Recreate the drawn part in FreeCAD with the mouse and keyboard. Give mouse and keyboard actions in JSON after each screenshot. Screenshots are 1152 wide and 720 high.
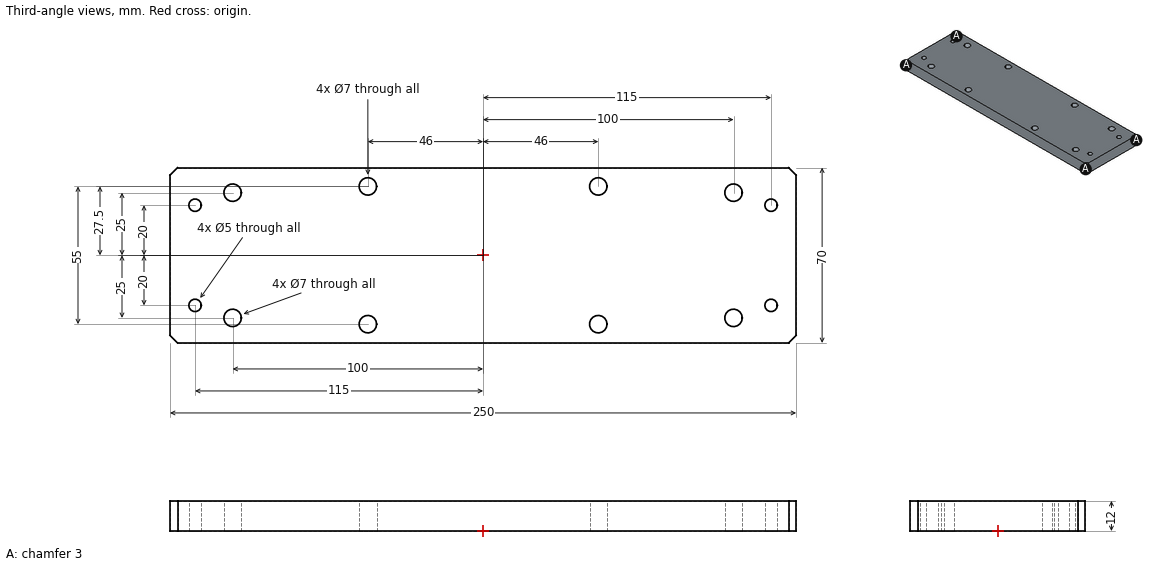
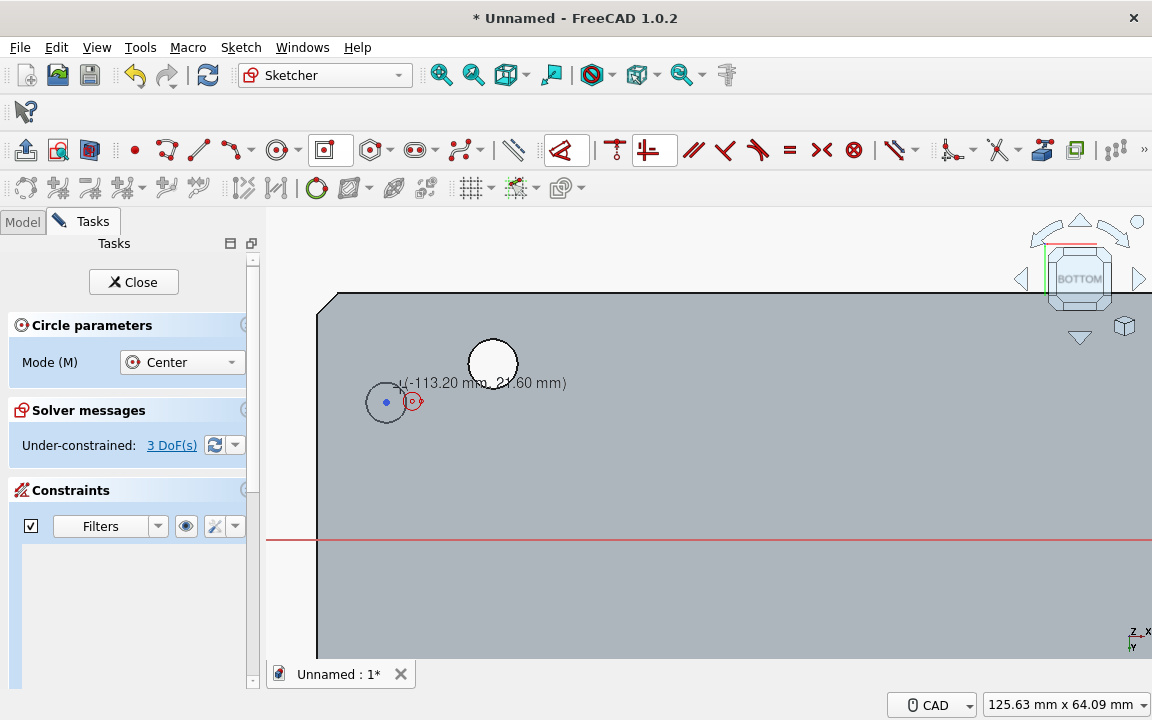
{"action": "scroll", "coordinate": [400, 387], "scroll_direction": "down", "scroll_amount": 6}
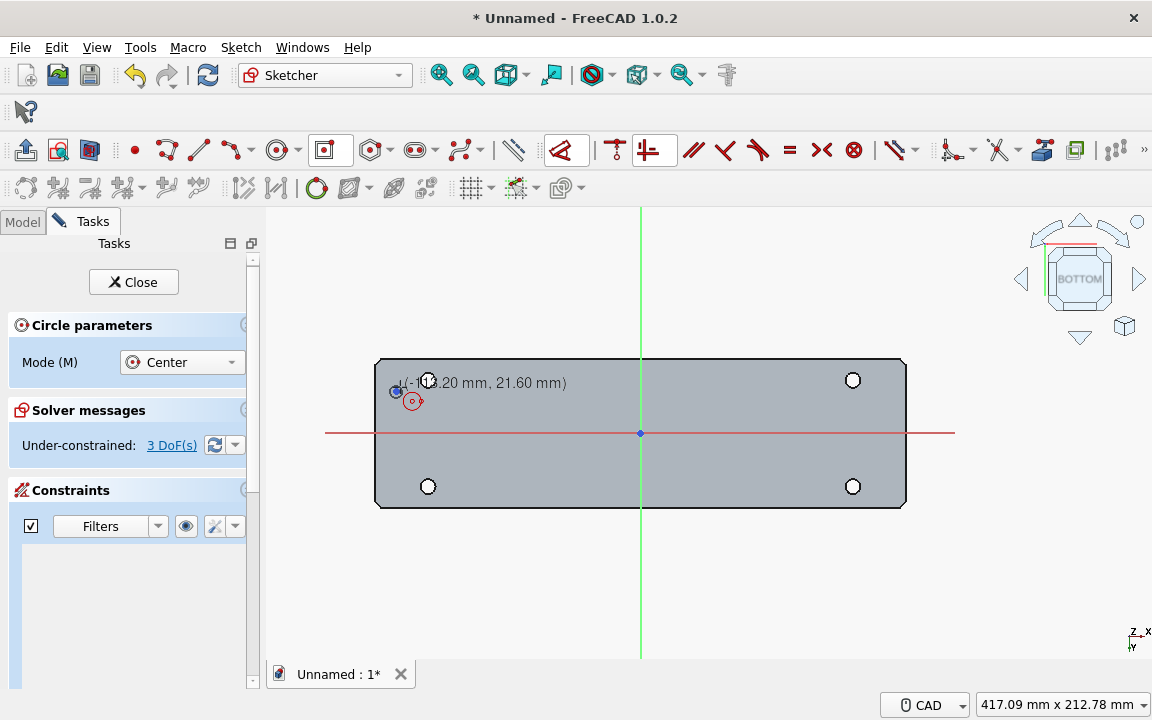
{"action": "scroll", "coordinate": [396, 476], "scroll_direction": "up", "scroll_amount": 8}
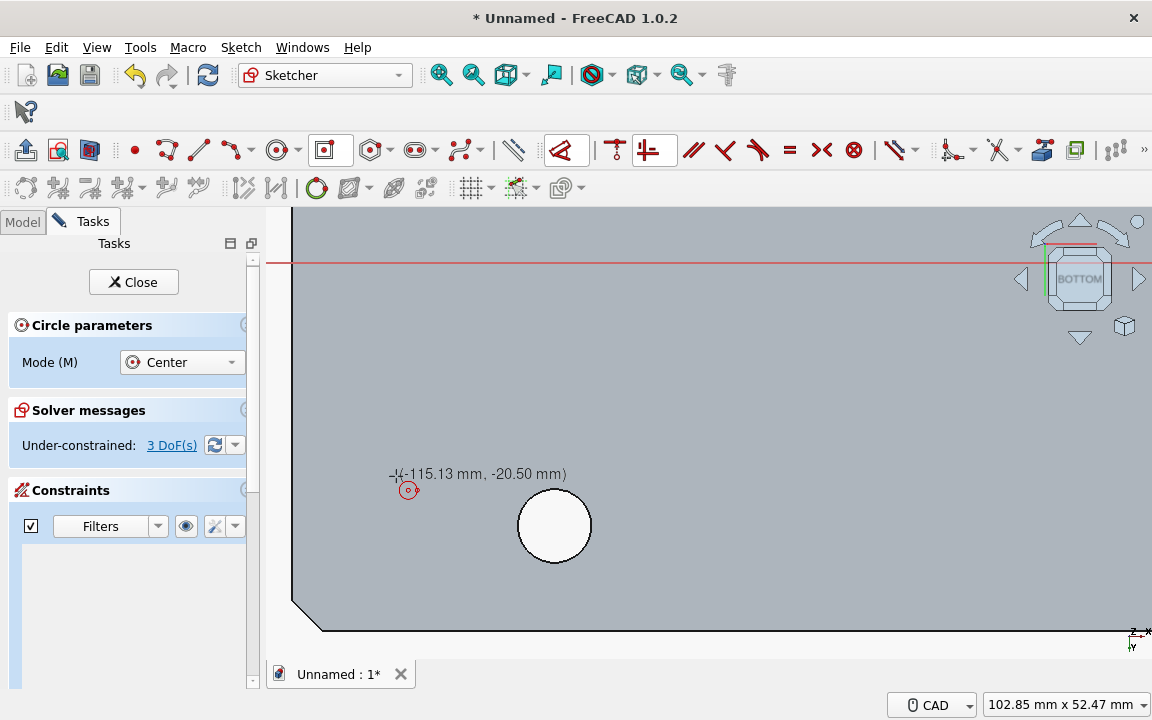
{"action": "scroll", "coordinate": [396, 476], "scroll_direction": "down", "scroll_amount": 8}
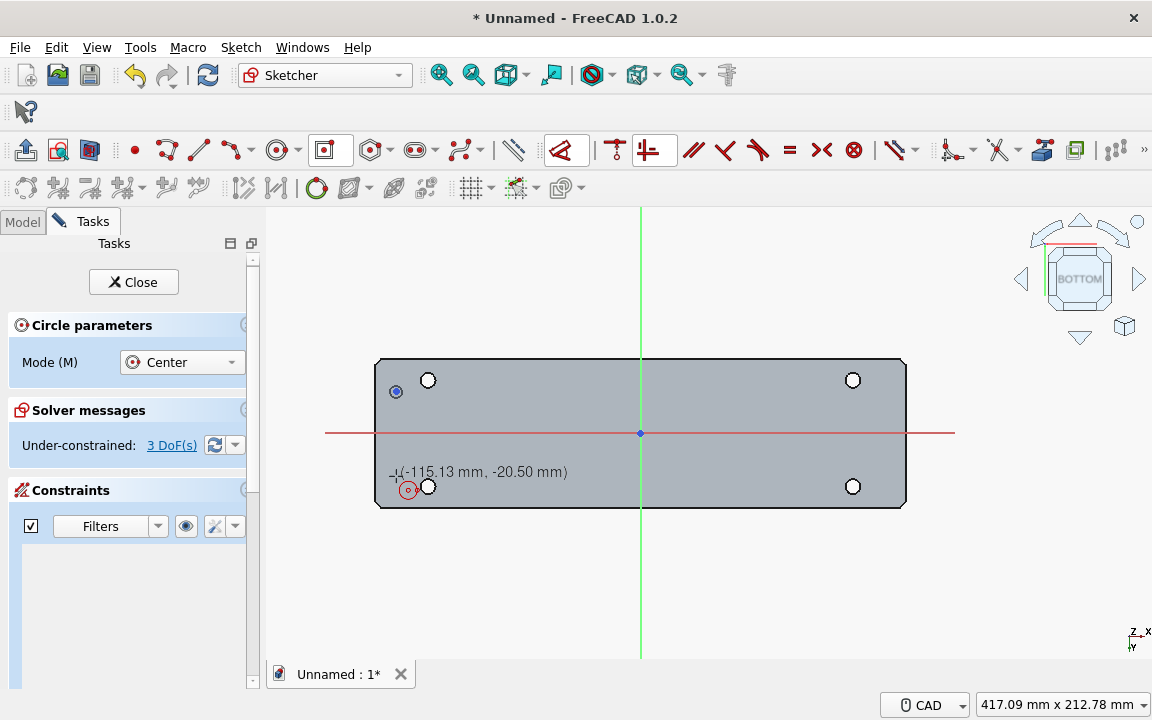
{"action": "left_click", "coordinate": [396, 476]}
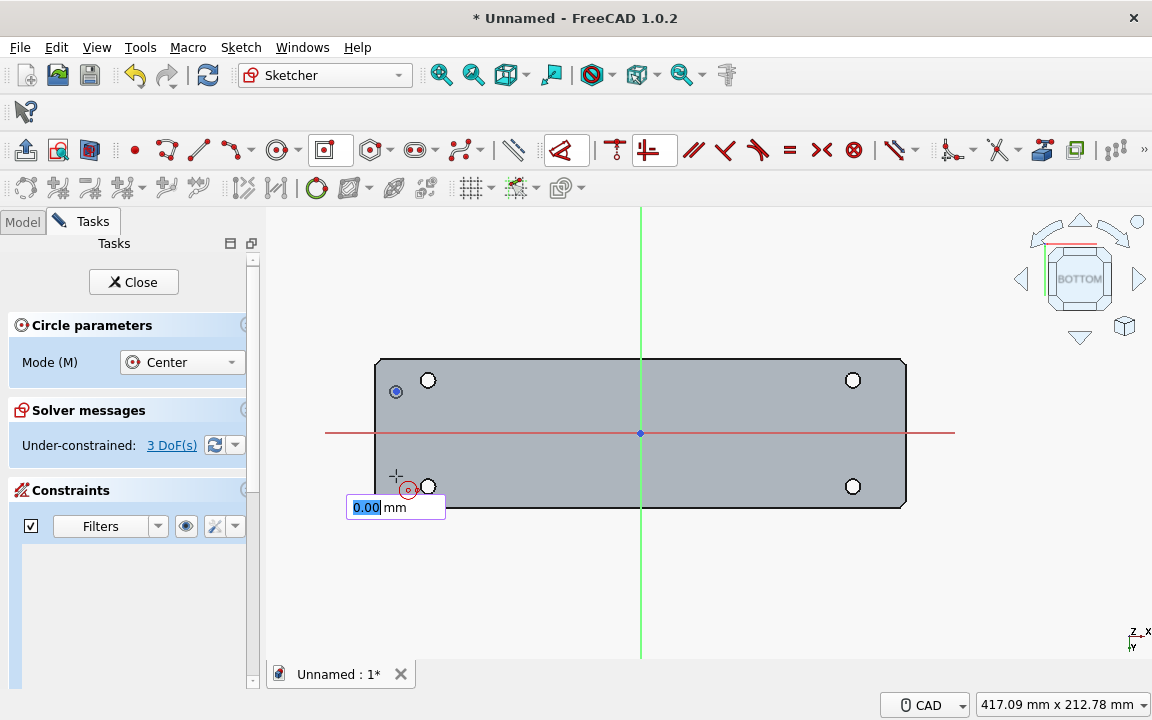
{"action": "scroll", "coordinate": [400, 472], "scroll_direction": "up", "scroll_amount": 6}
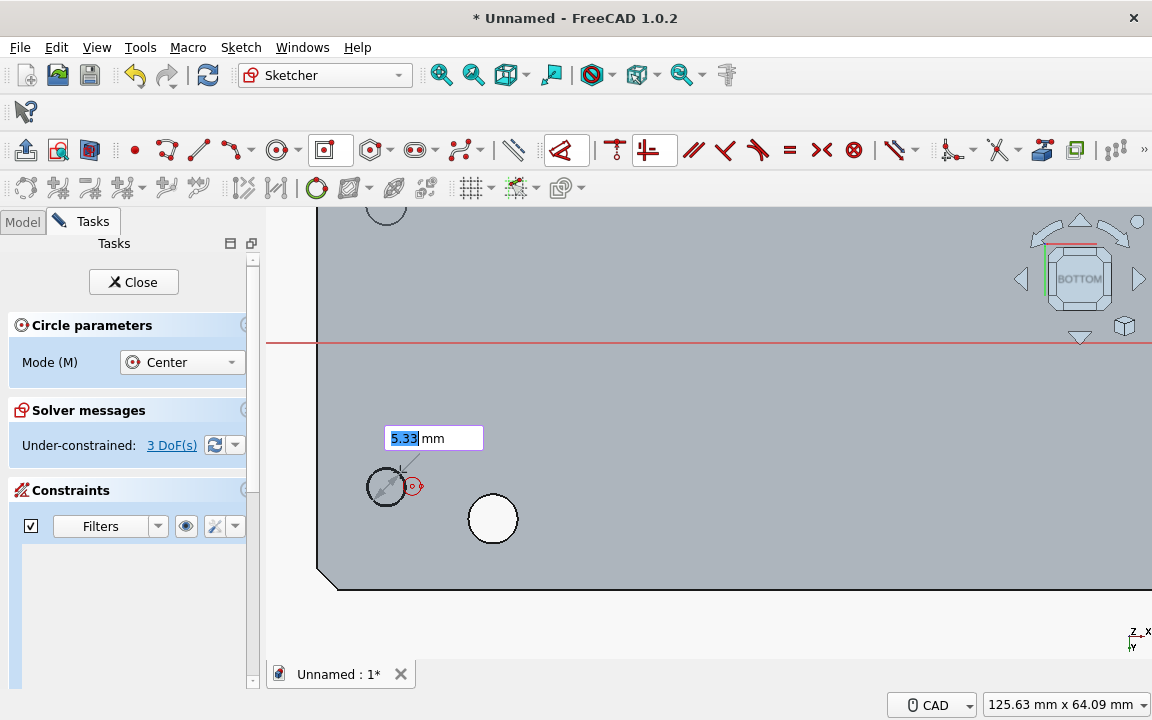
{"action": "left_click", "coordinate": [400, 471]}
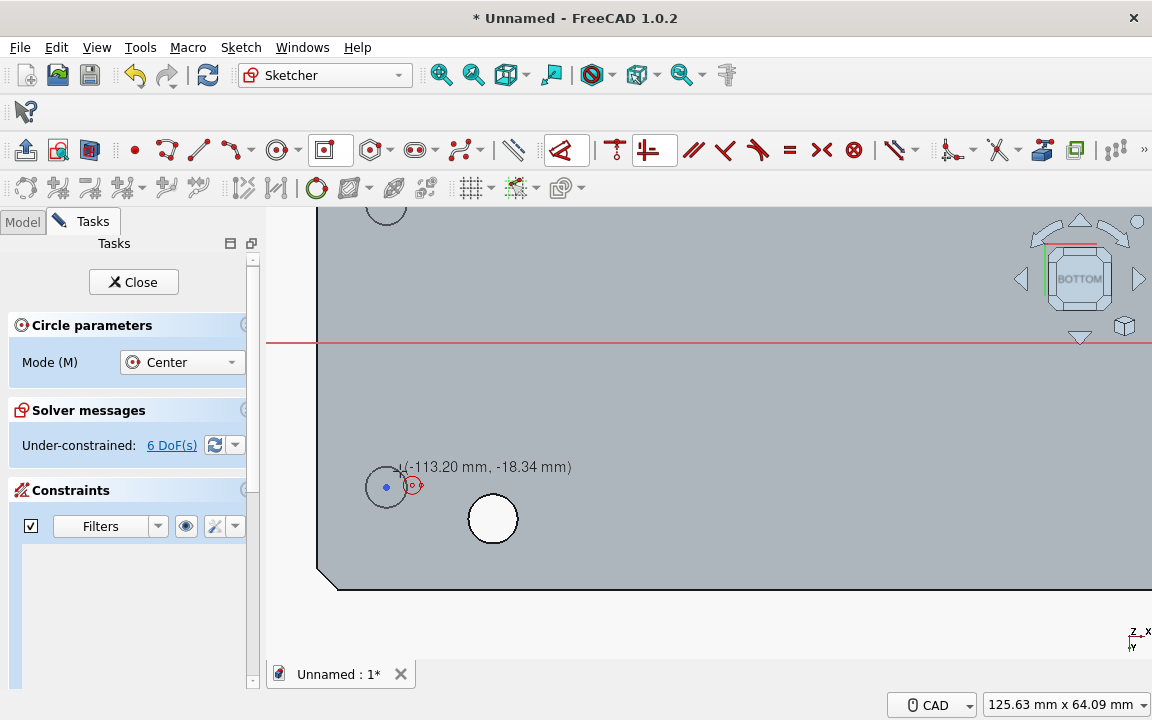
{"action": "scroll", "coordinate": [400, 472], "scroll_direction": "down", "scroll_amount": 6}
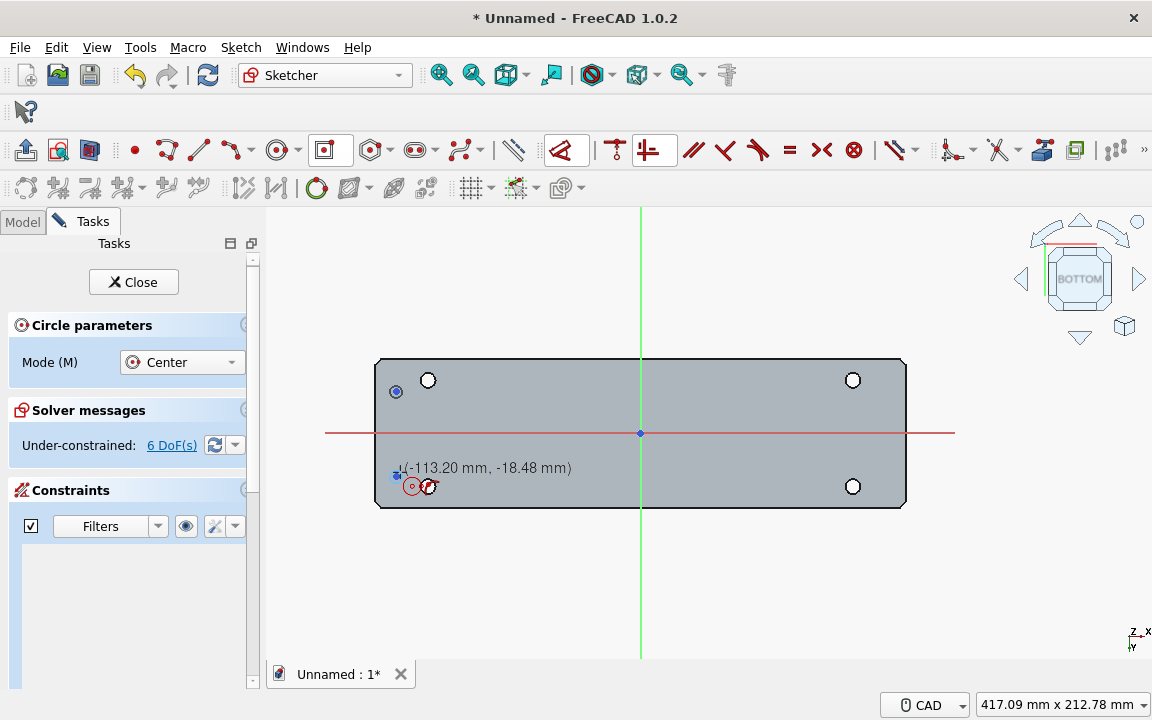
{"action": "scroll", "coordinate": [885, 476], "scroll_direction": "up", "scroll_amount": 8}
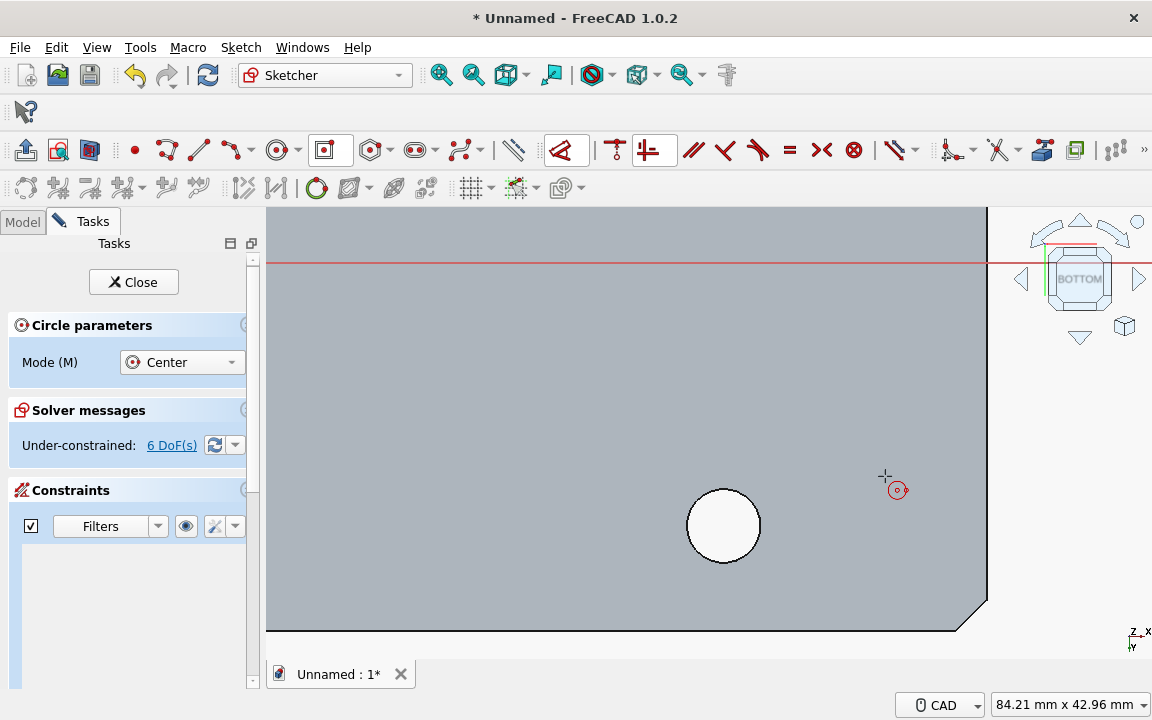
{"action": "scroll", "coordinate": [886, 476], "scroll_direction": "down", "scroll_amount": 8}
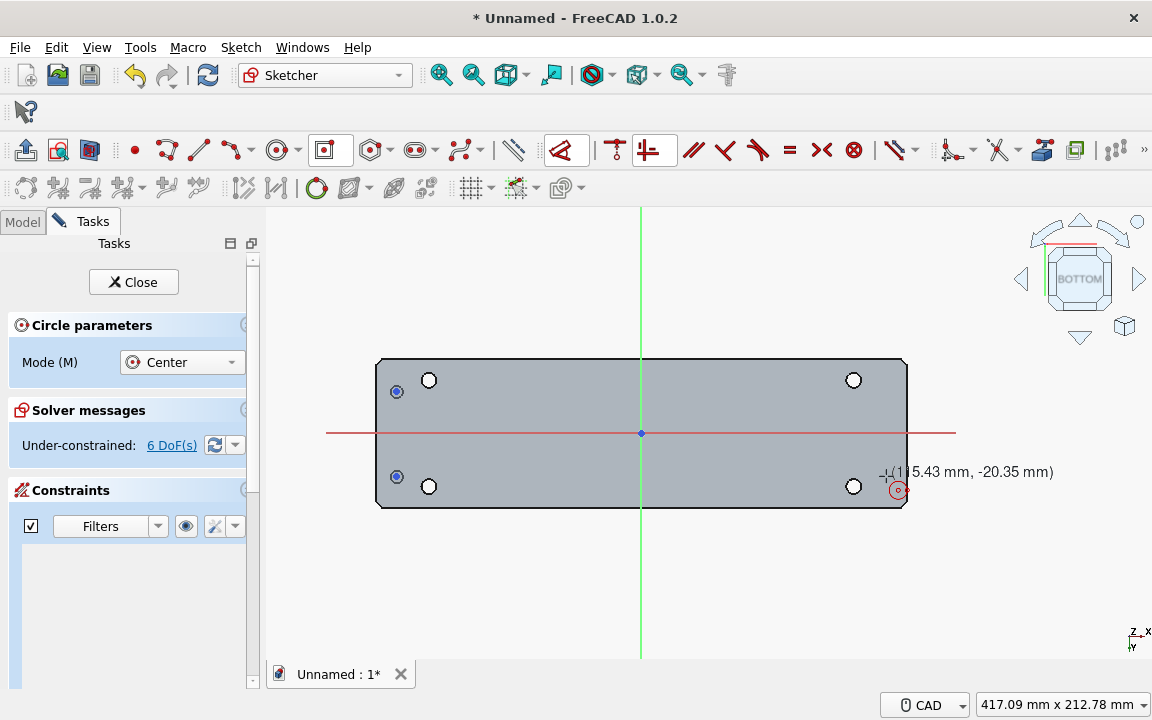
{"action": "left_click", "coordinate": [886, 476]}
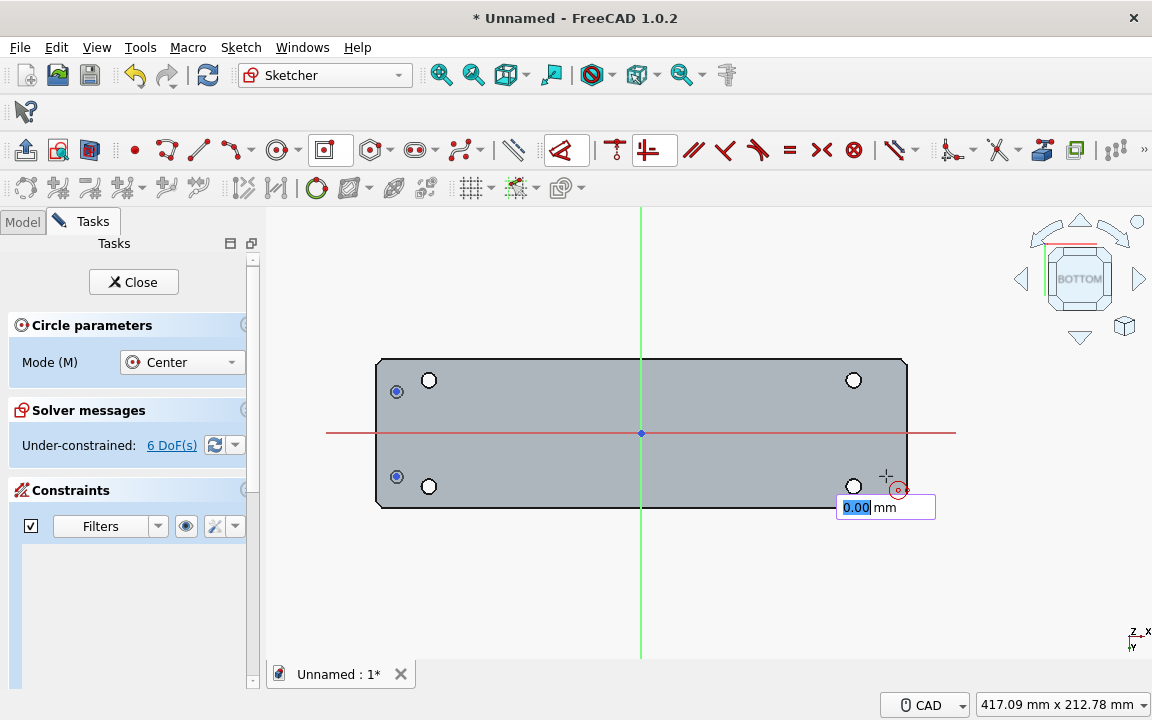
{"action": "scroll", "coordinate": [889, 472], "scroll_direction": "up", "scroll_amount": 6}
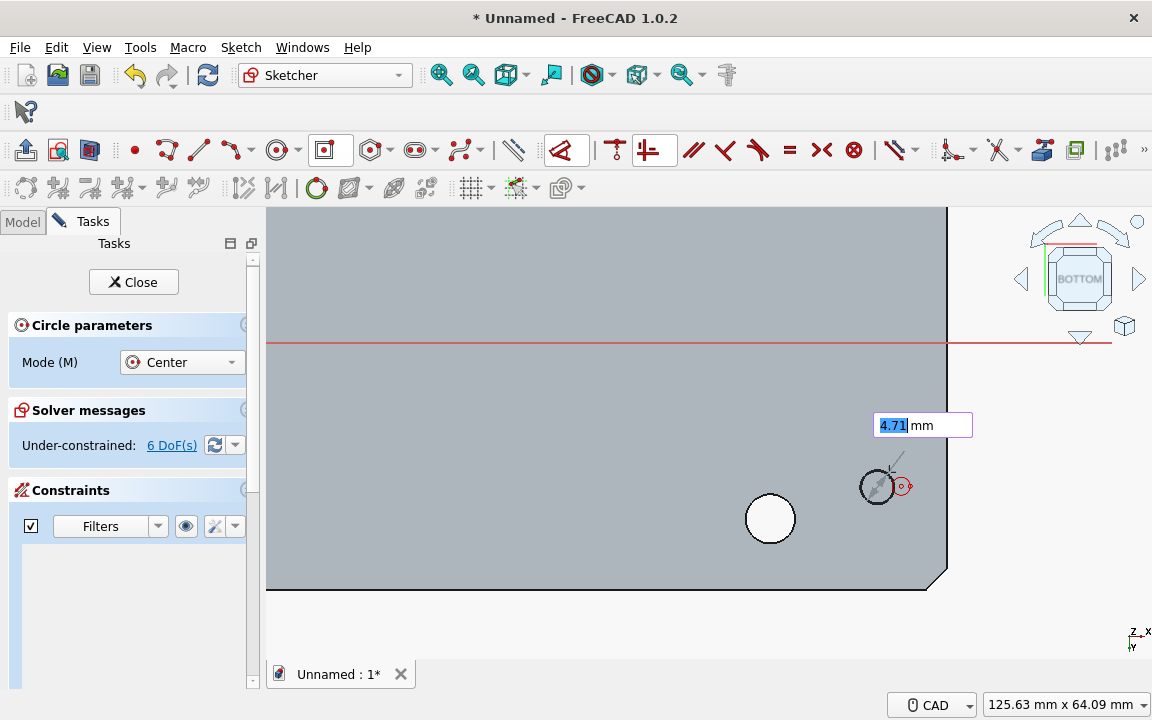
{"action": "left_click", "coordinate": [889, 471]}